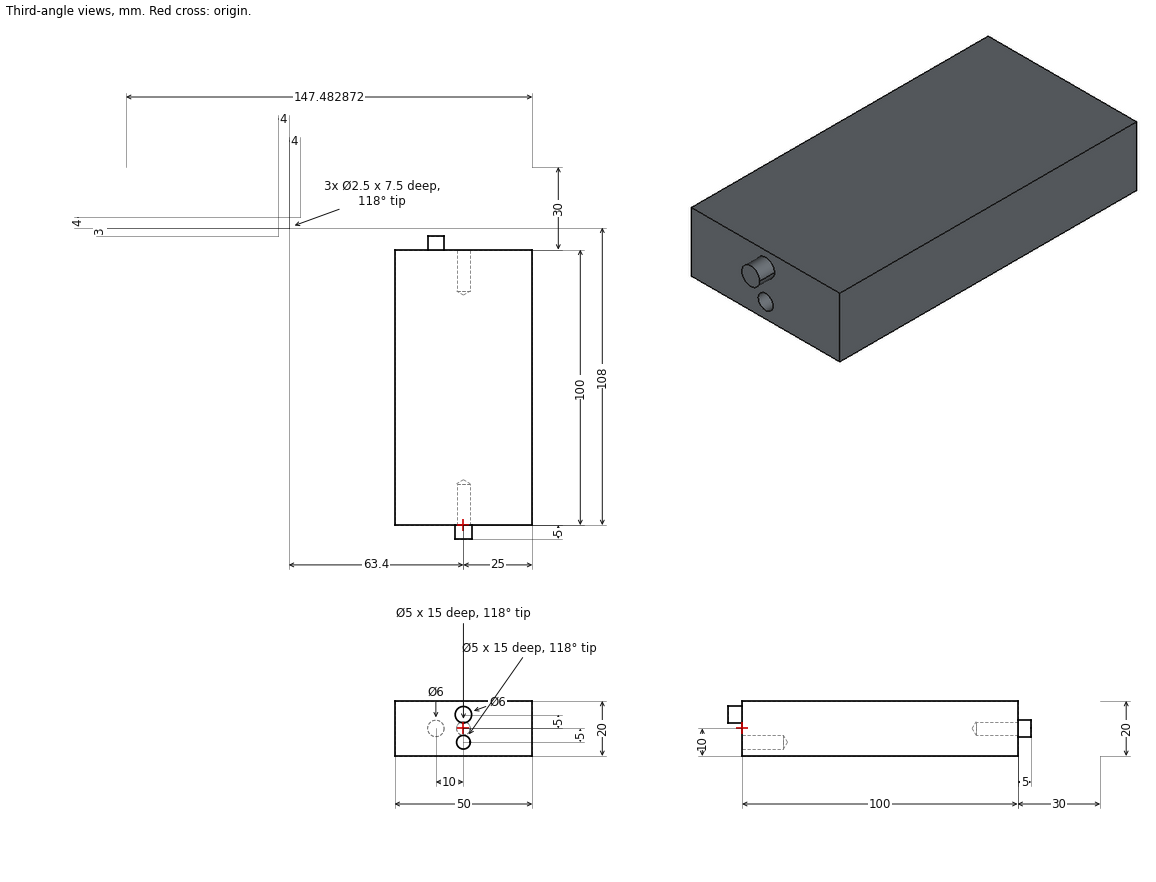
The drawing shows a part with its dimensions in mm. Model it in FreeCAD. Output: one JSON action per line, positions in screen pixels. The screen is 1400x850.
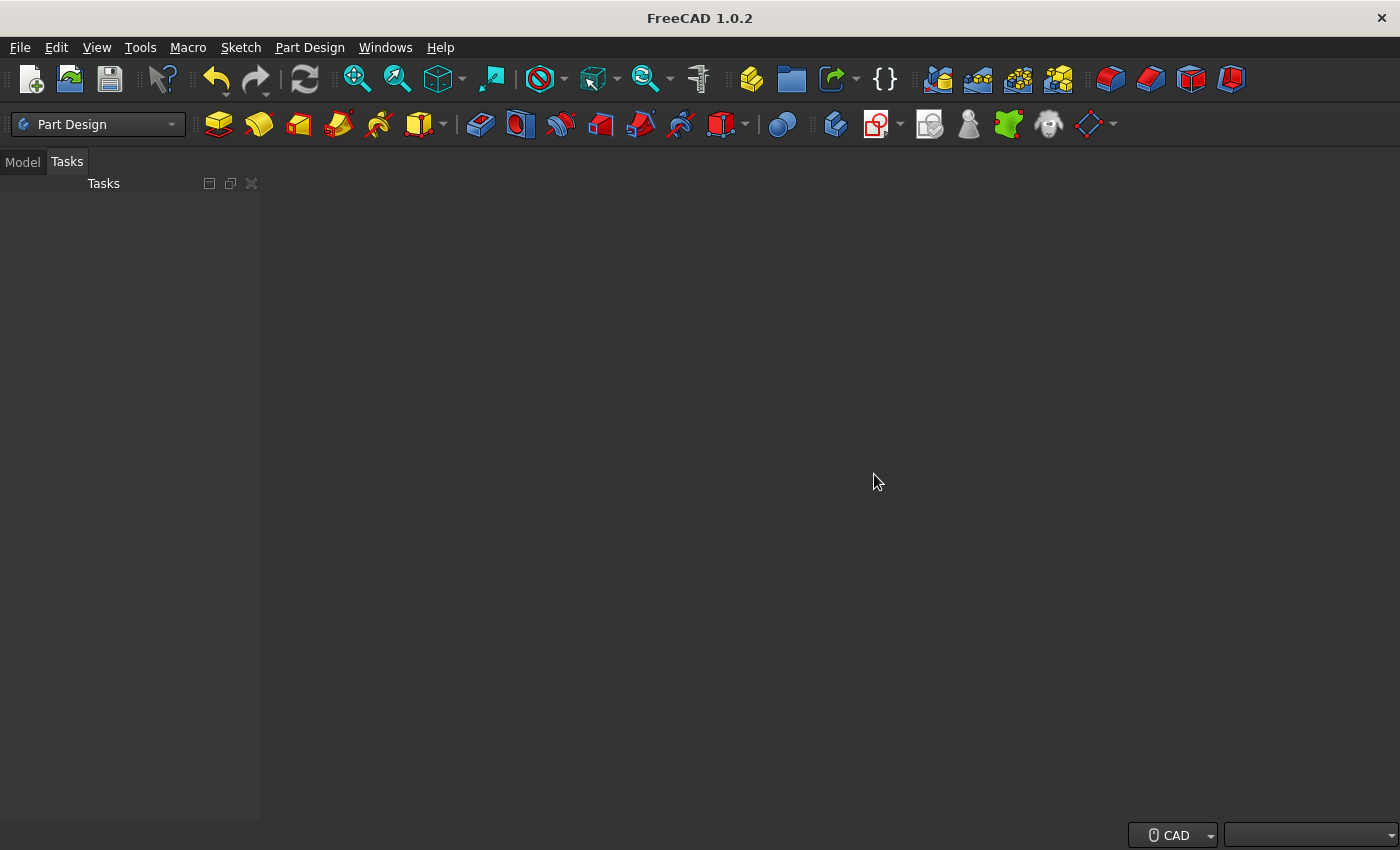
{"action": "left_click", "coordinate": [30, 80]}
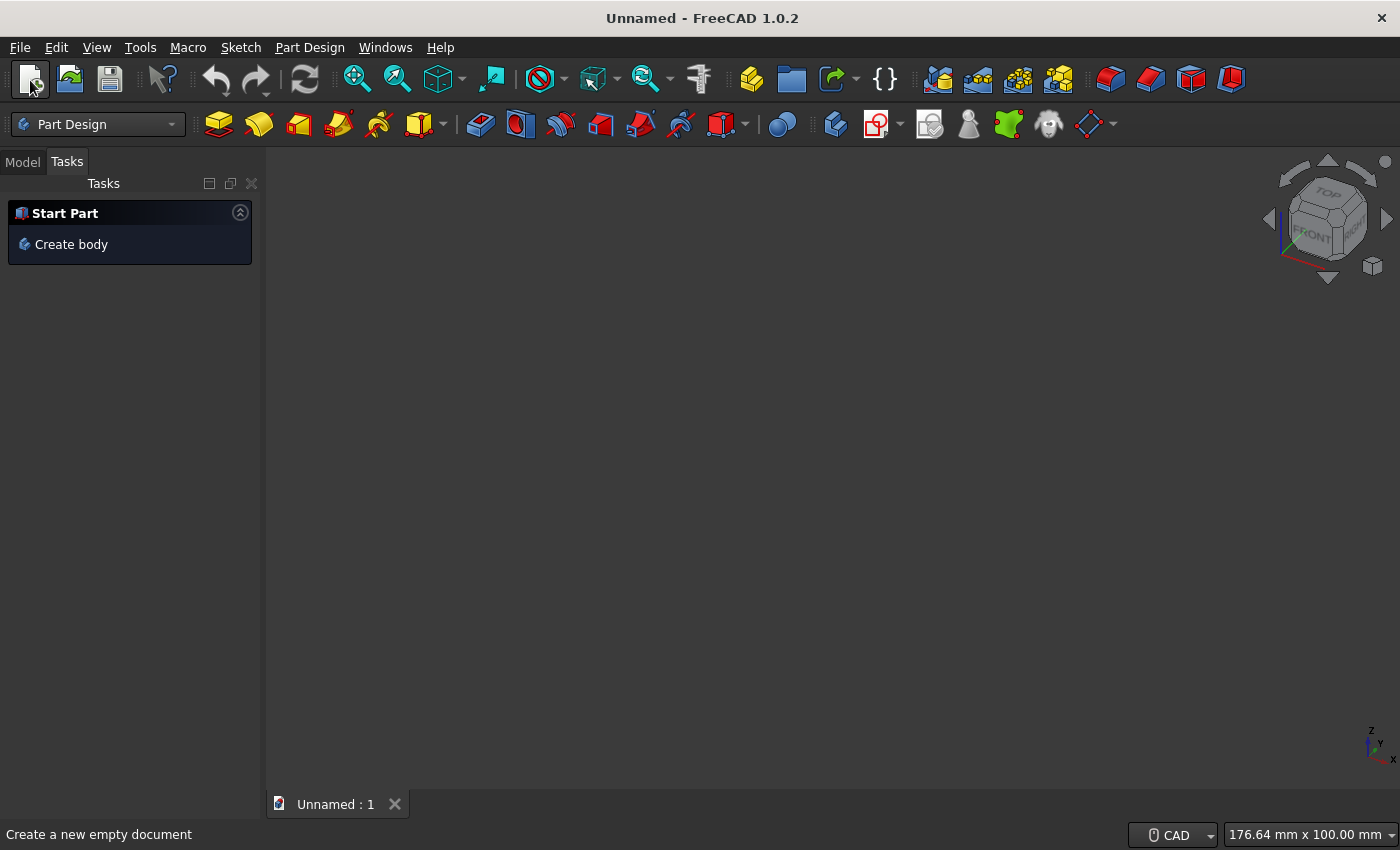
{"action": "left_click", "coordinate": [876, 124]}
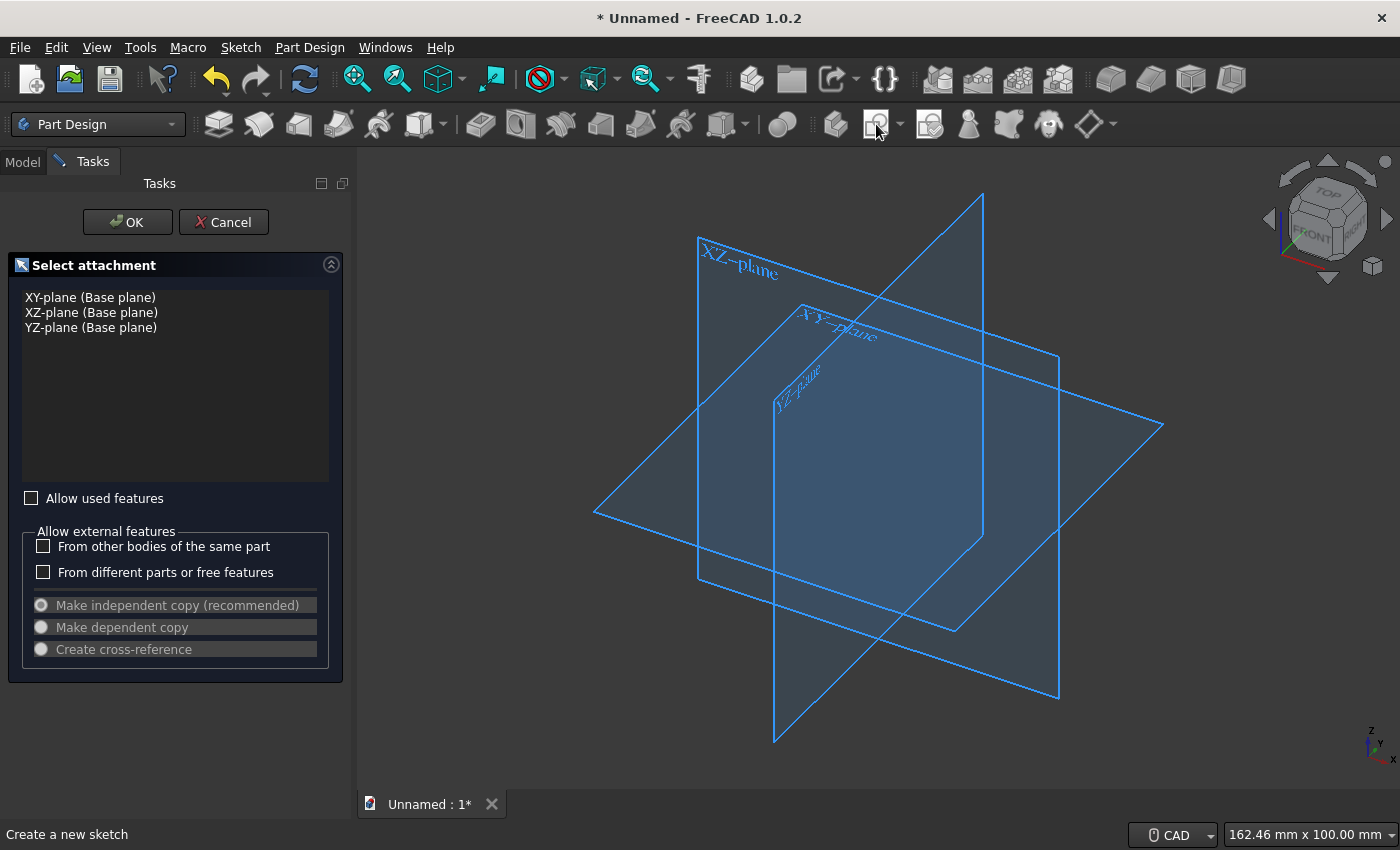
{"action": "left_click", "coordinate": [82, 312]}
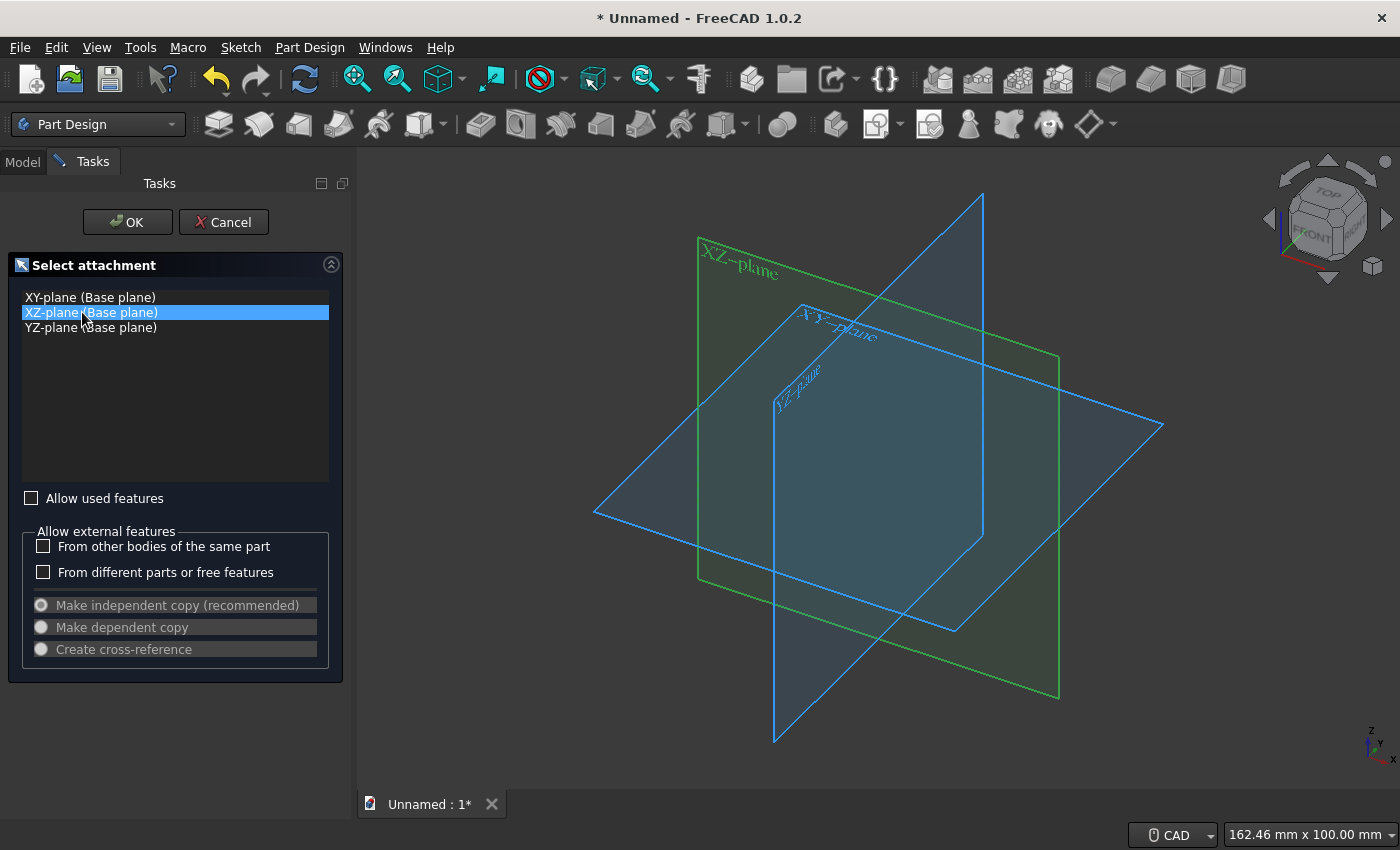
{"action": "left_click", "coordinate": [128, 222]}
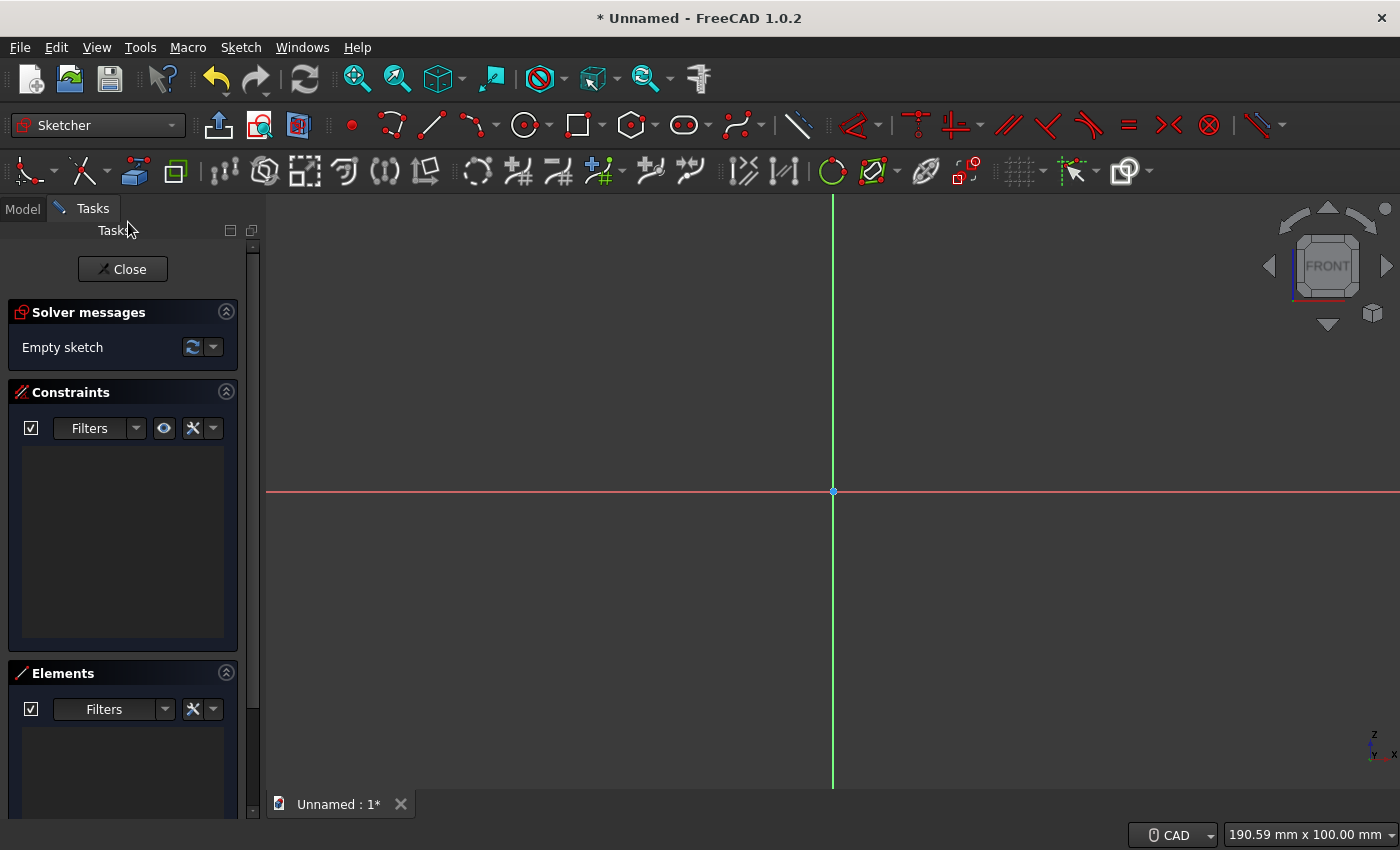
{"action": "scroll", "coordinate": [889, 491], "scroll_direction": "up", "scroll_amount": 4}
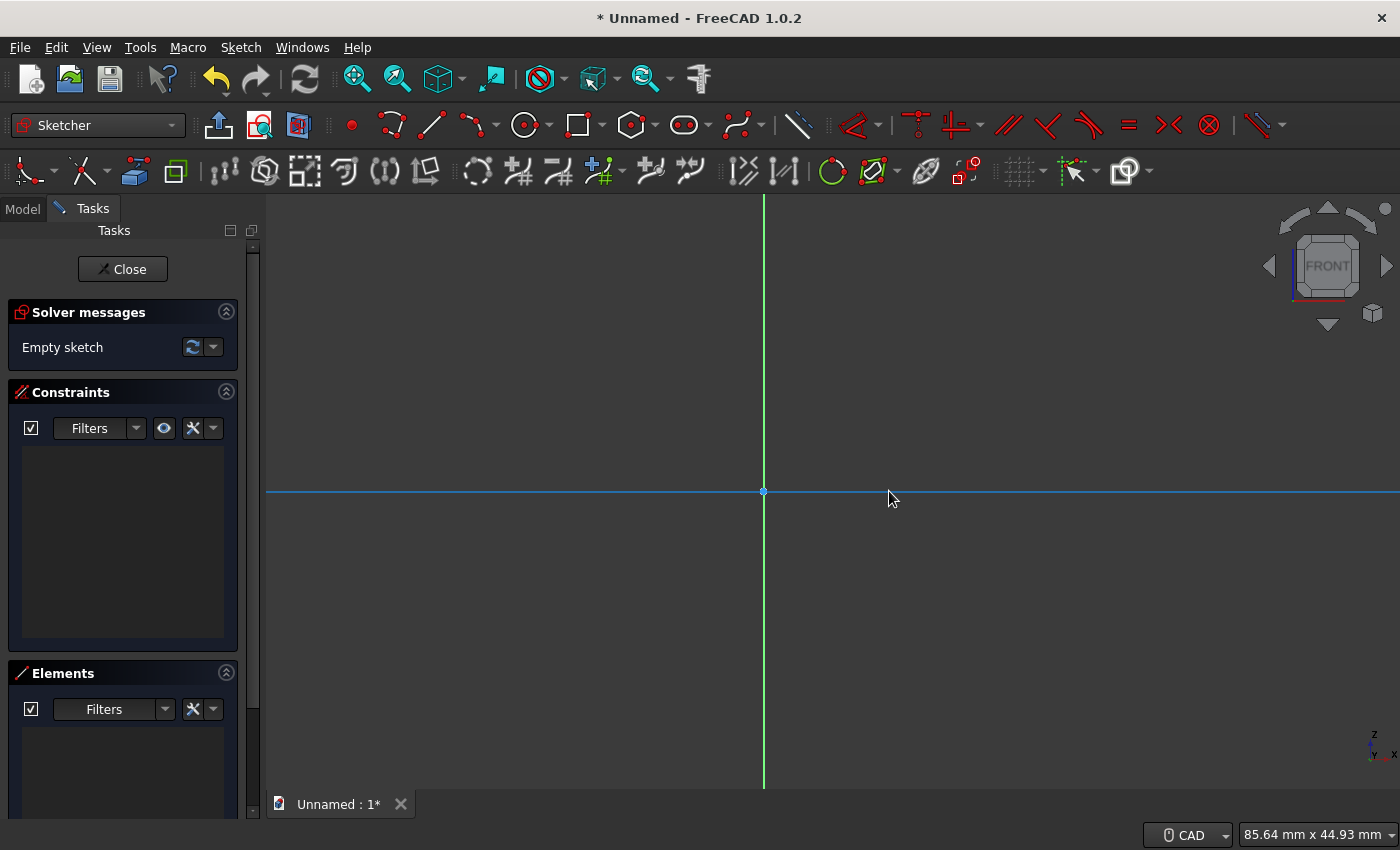
{"action": "key", "text": "g v"}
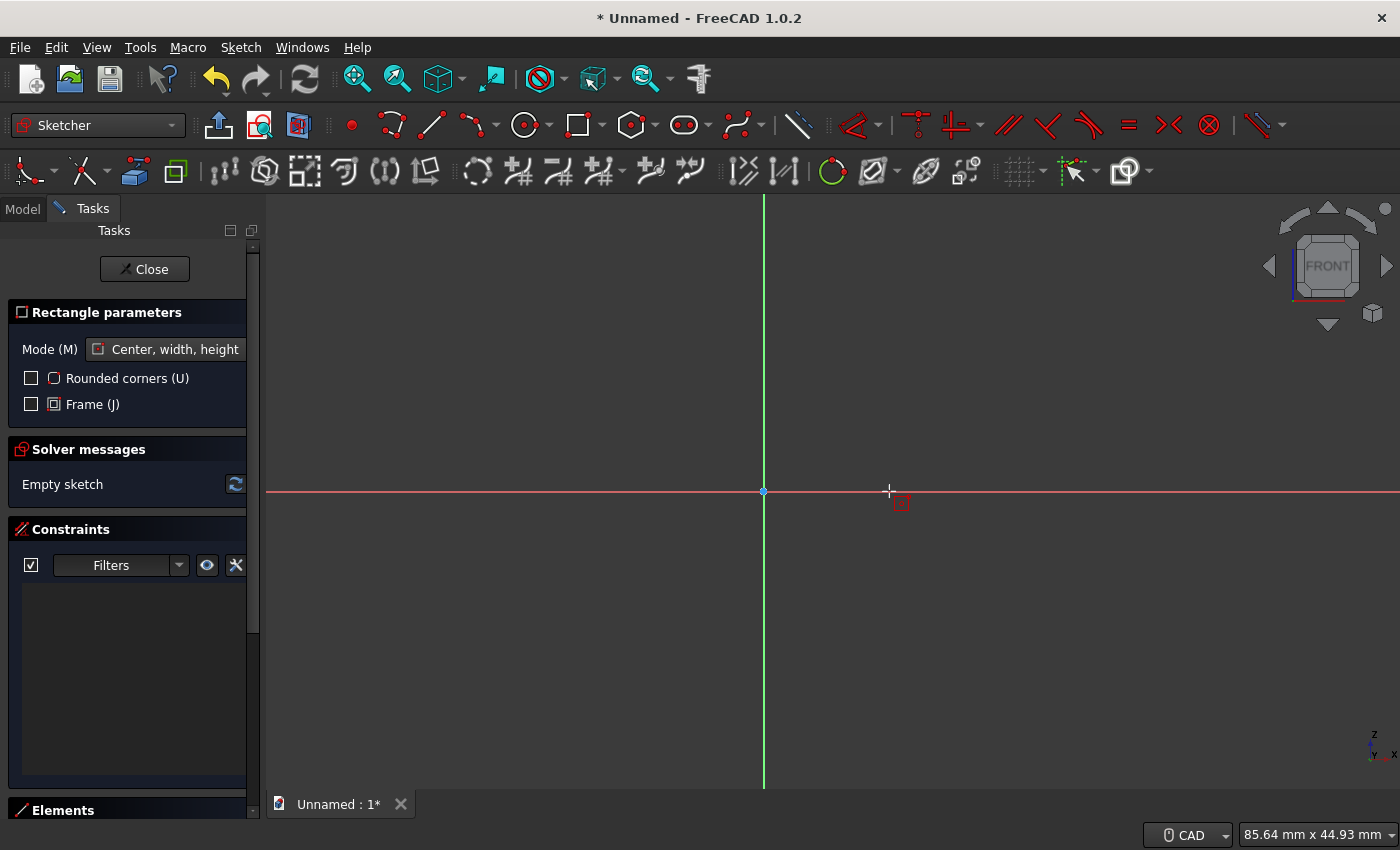
{"action": "left_click", "coordinate": [764, 492]}
{"action": "left_click", "coordinate": [1095, 359]}
{"action": "key", "text": "Escape"}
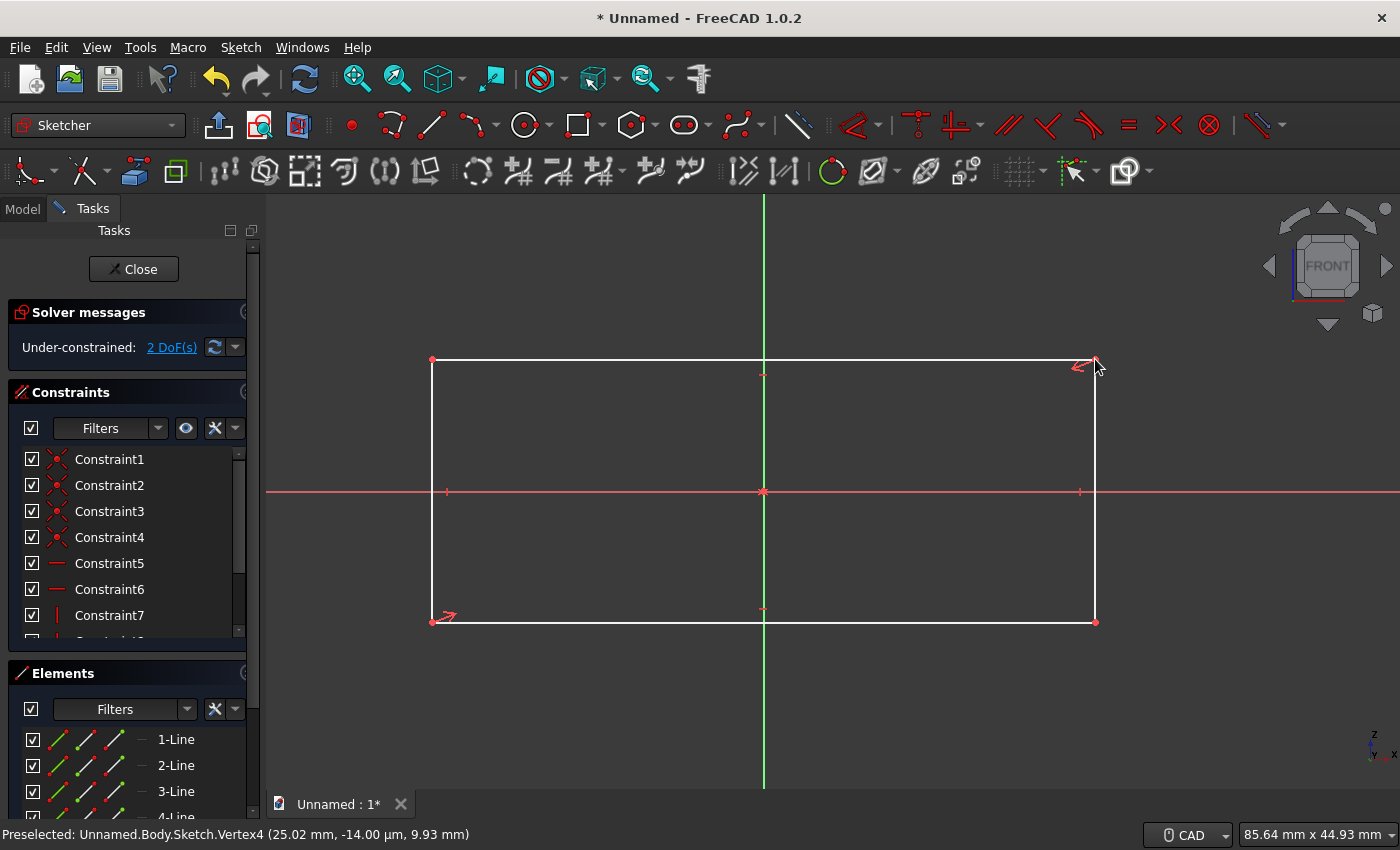
{"action": "left_click", "coordinate": [631, 623]}